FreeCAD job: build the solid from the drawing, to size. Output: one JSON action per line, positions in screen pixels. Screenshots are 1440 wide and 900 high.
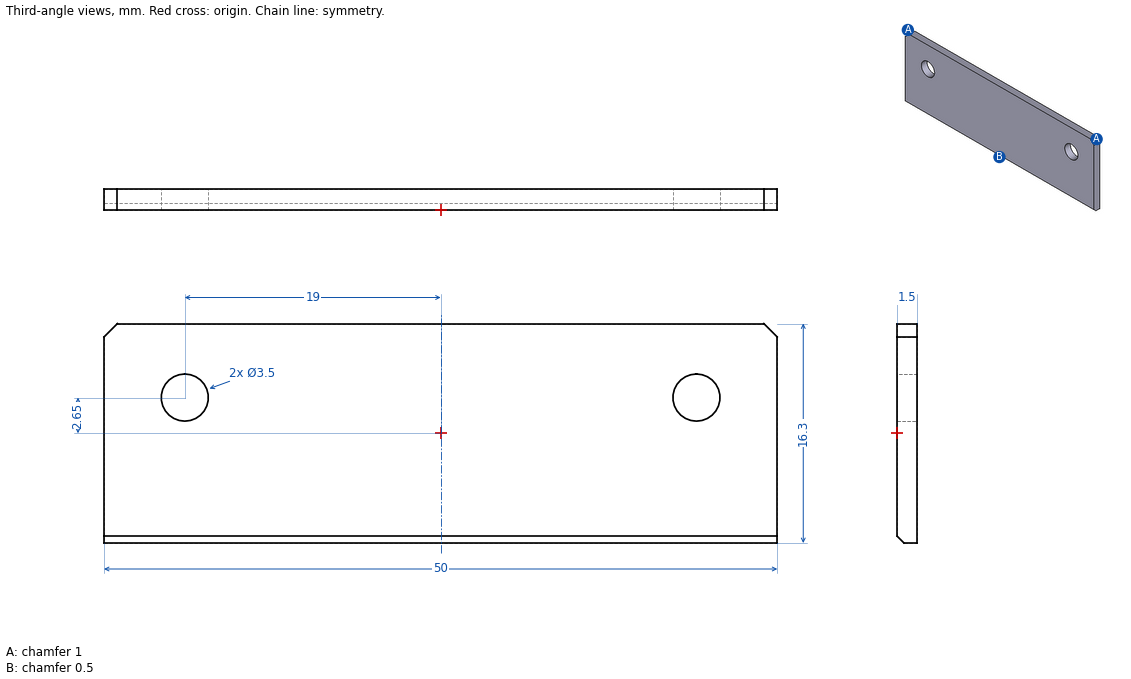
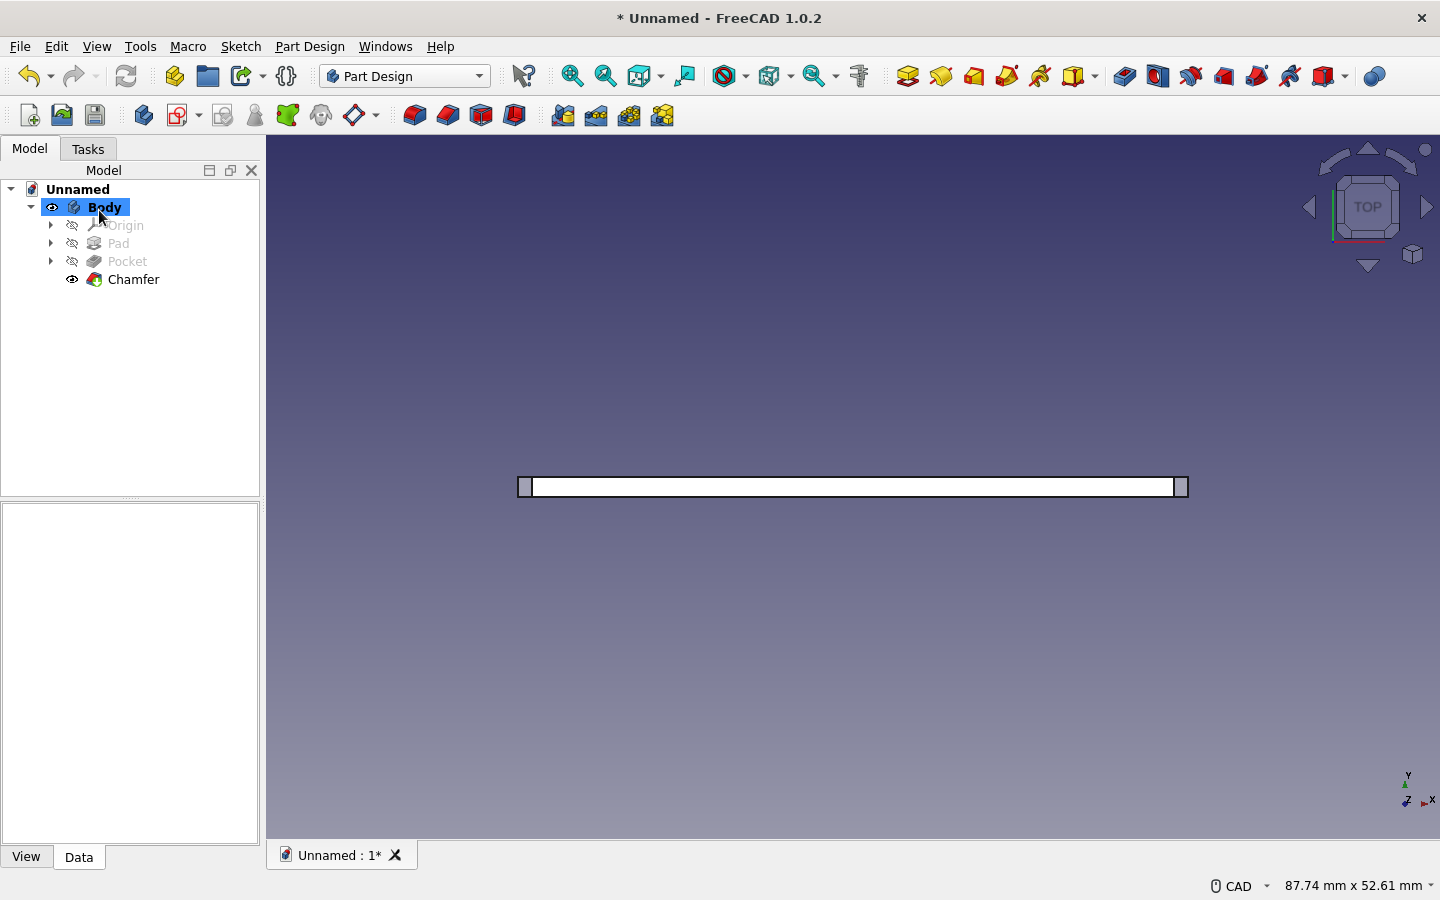
{"action": "key", "text": "1"}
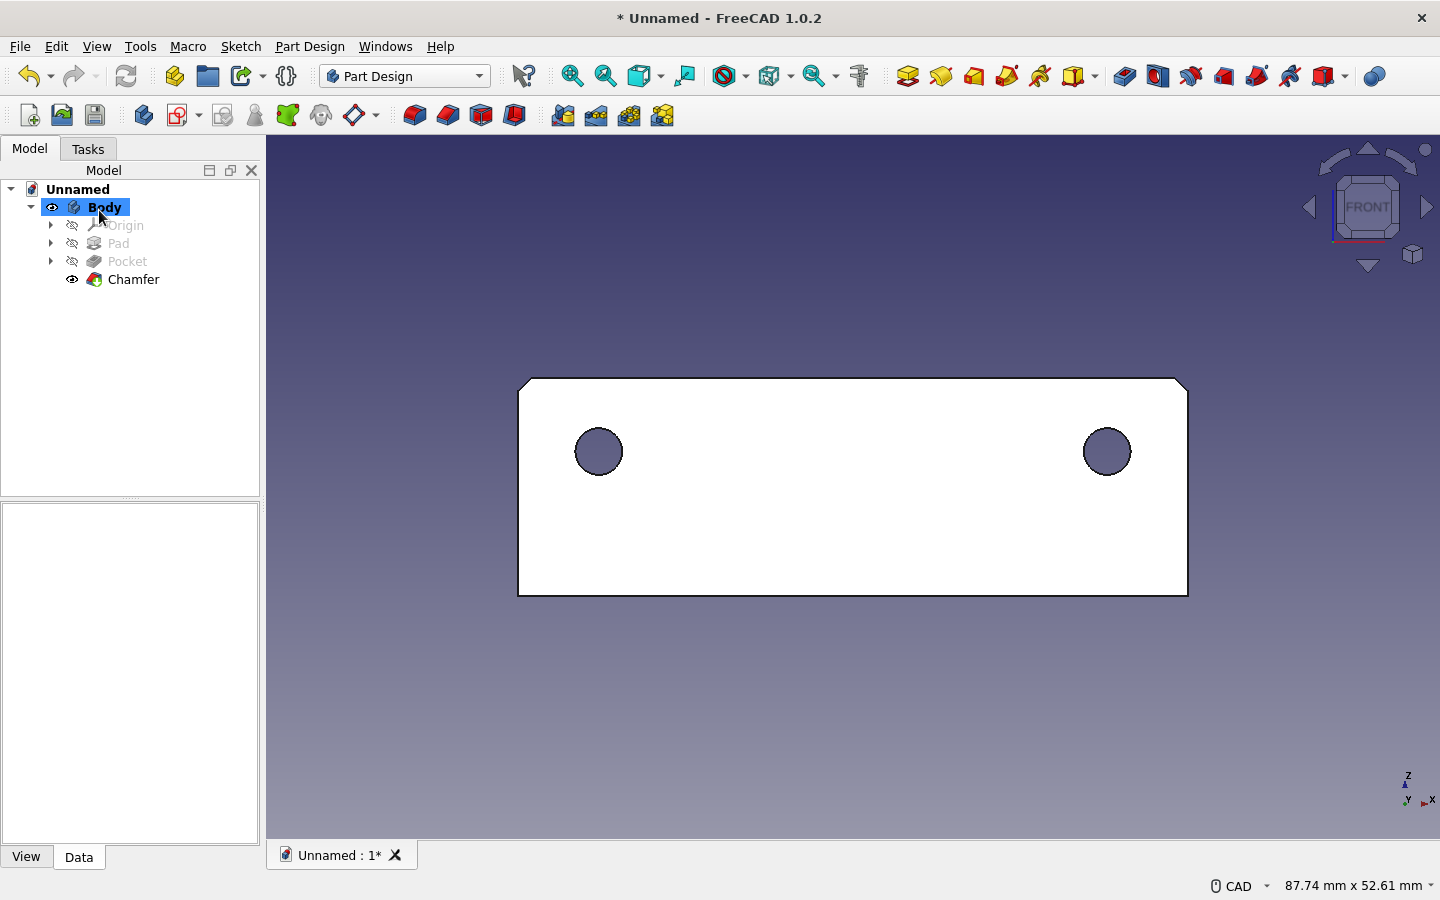
{"action": "key", "text": "3"}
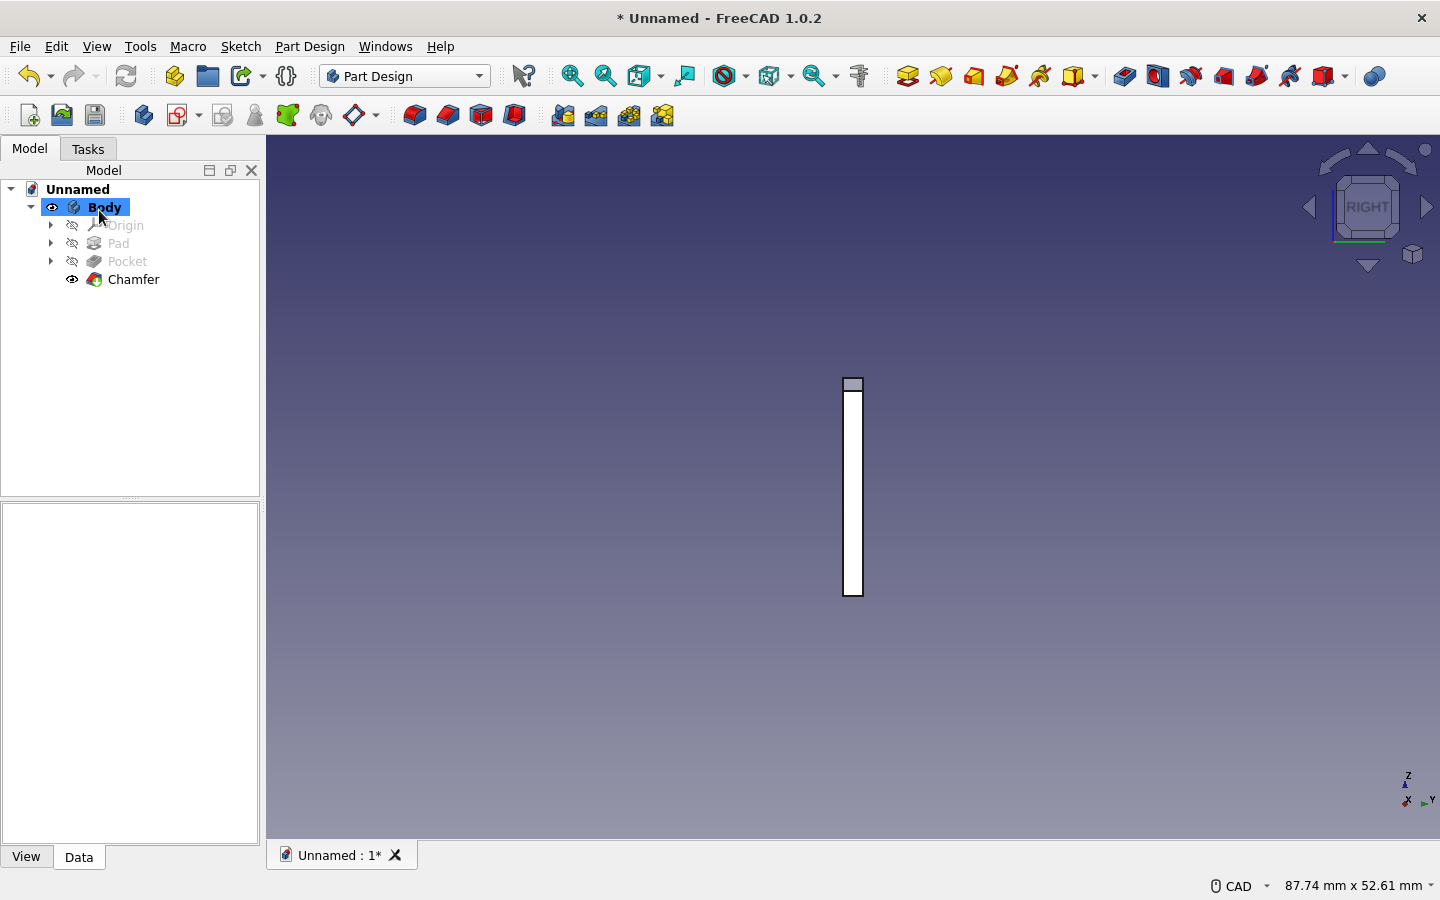
{"action": "key", "text": "v f"}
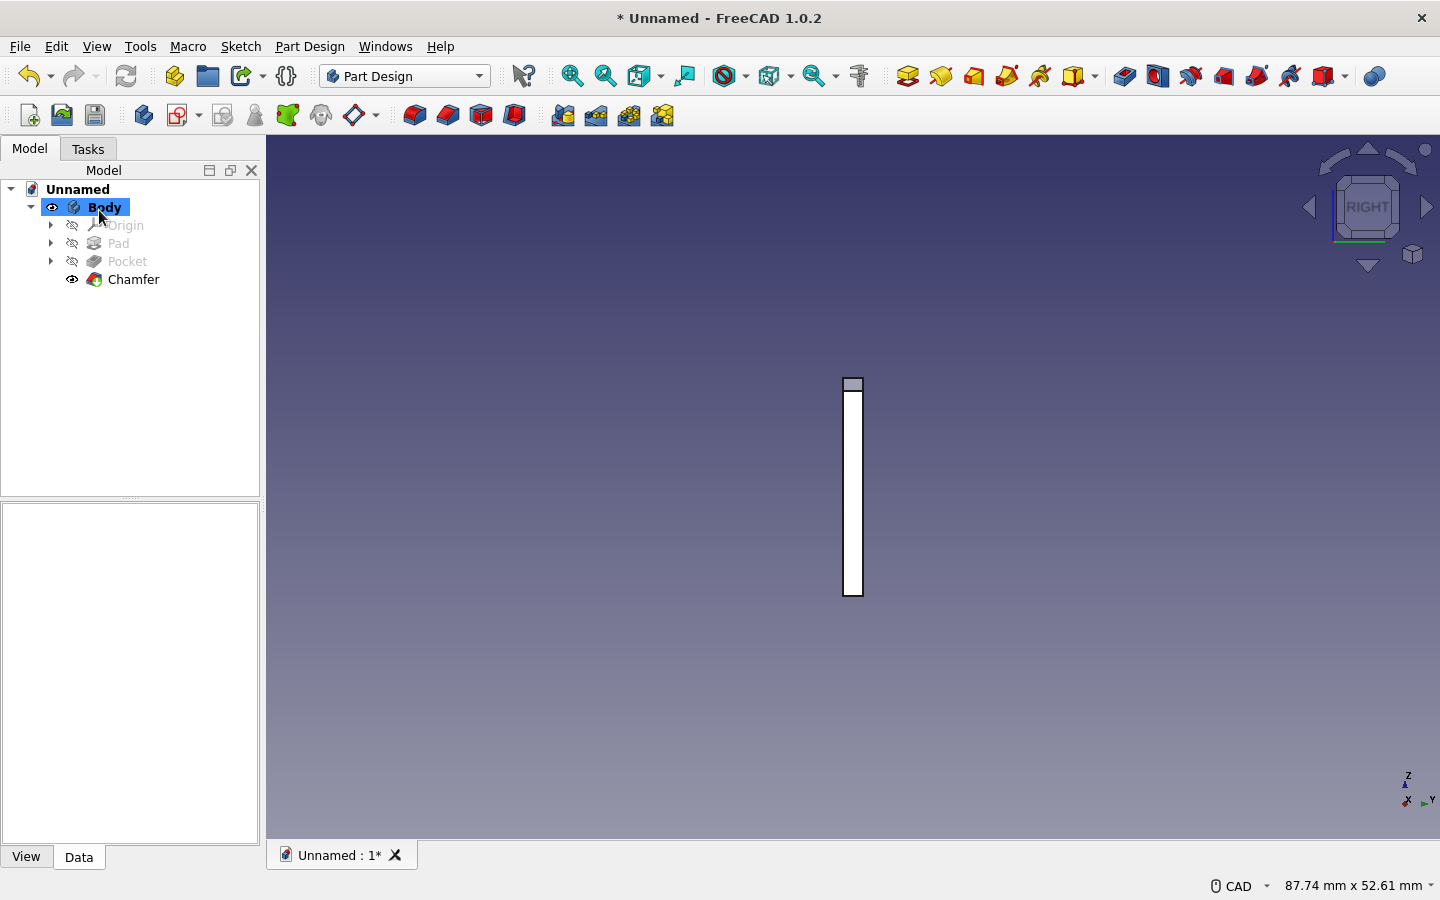
{"action": "key", "text": "5"}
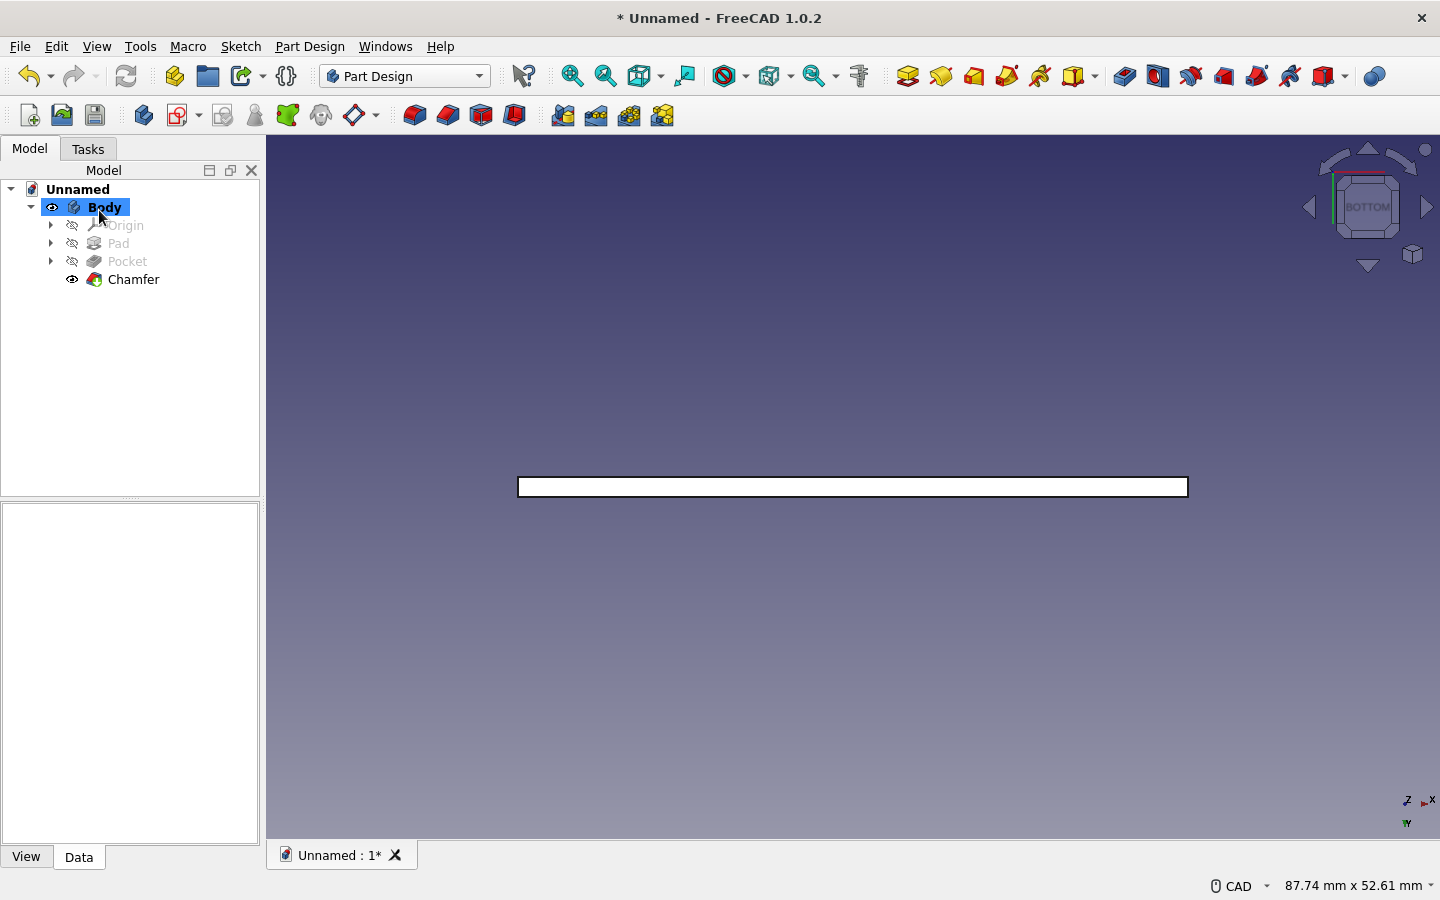
{"action": "left_click", "coordinate": [853, 476]}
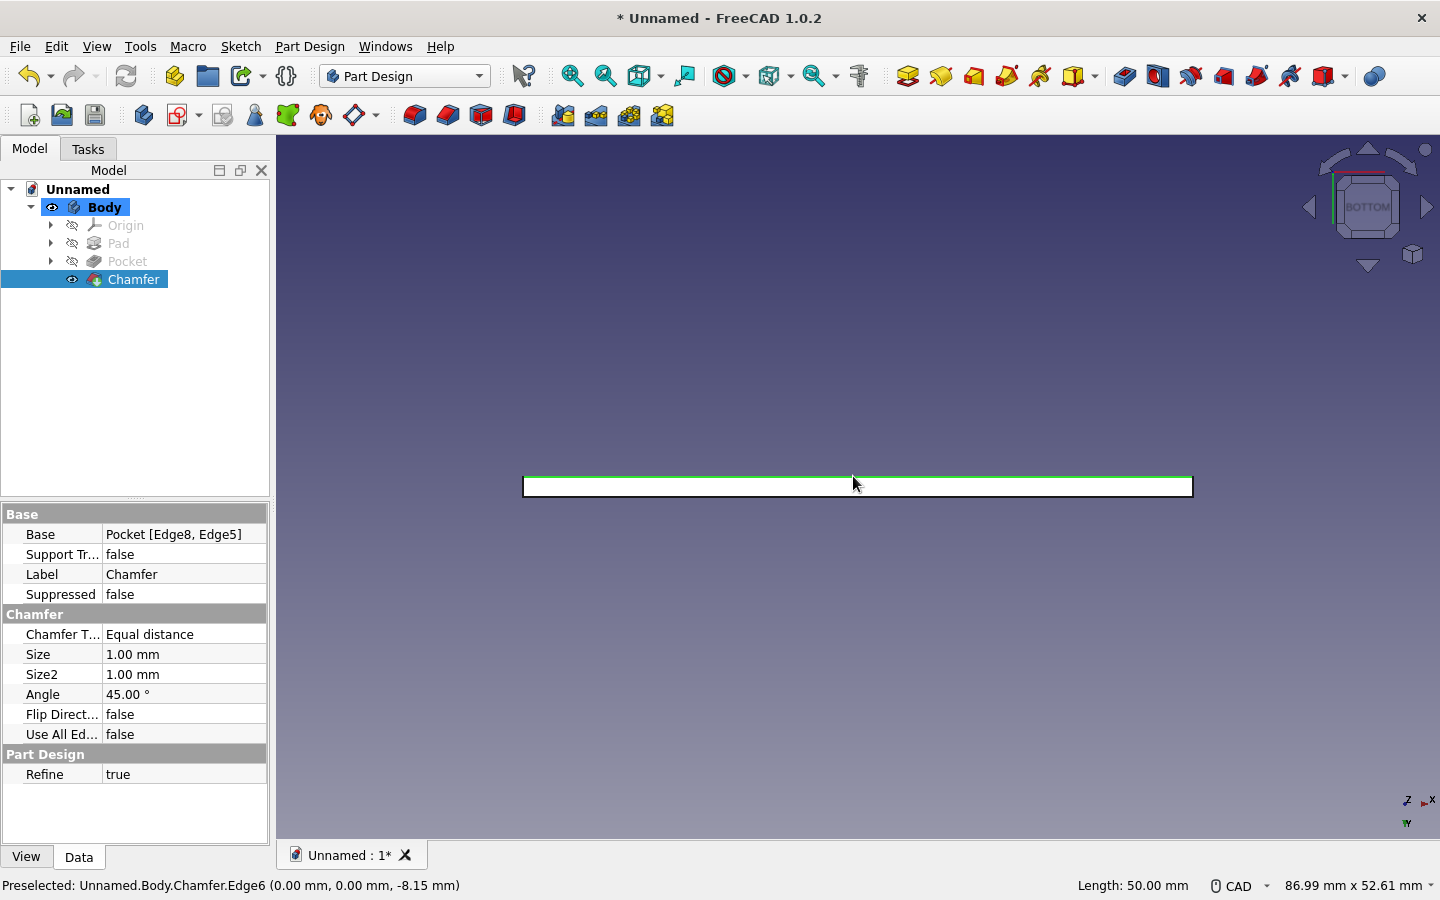
{"action": "left_click", "coordinate": [448, 116]}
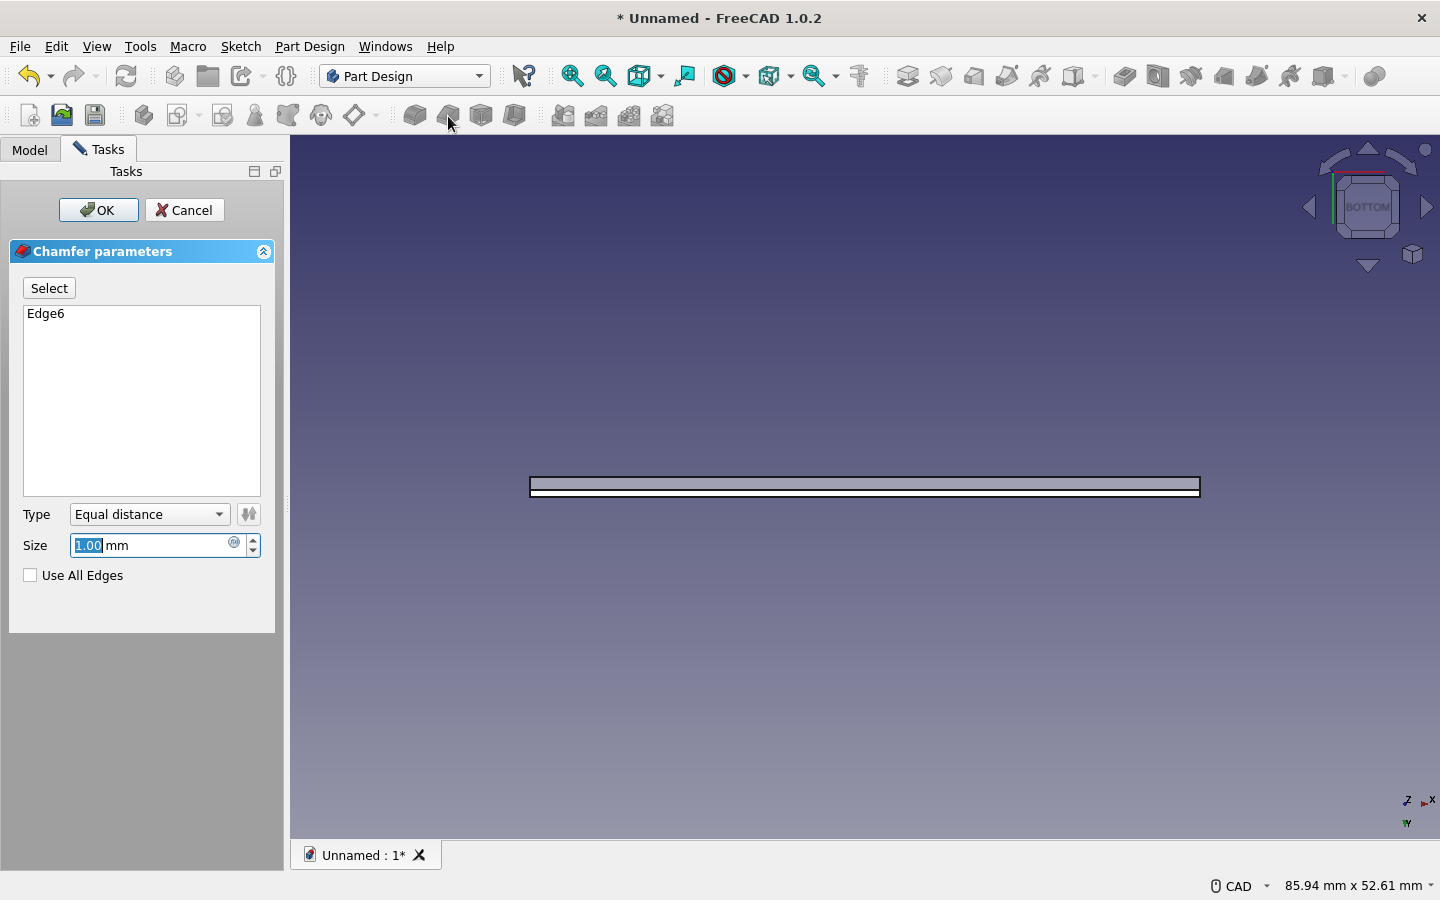
{"action": "type", "text": "0.5"}
{"action": "key", "text": "Tab"}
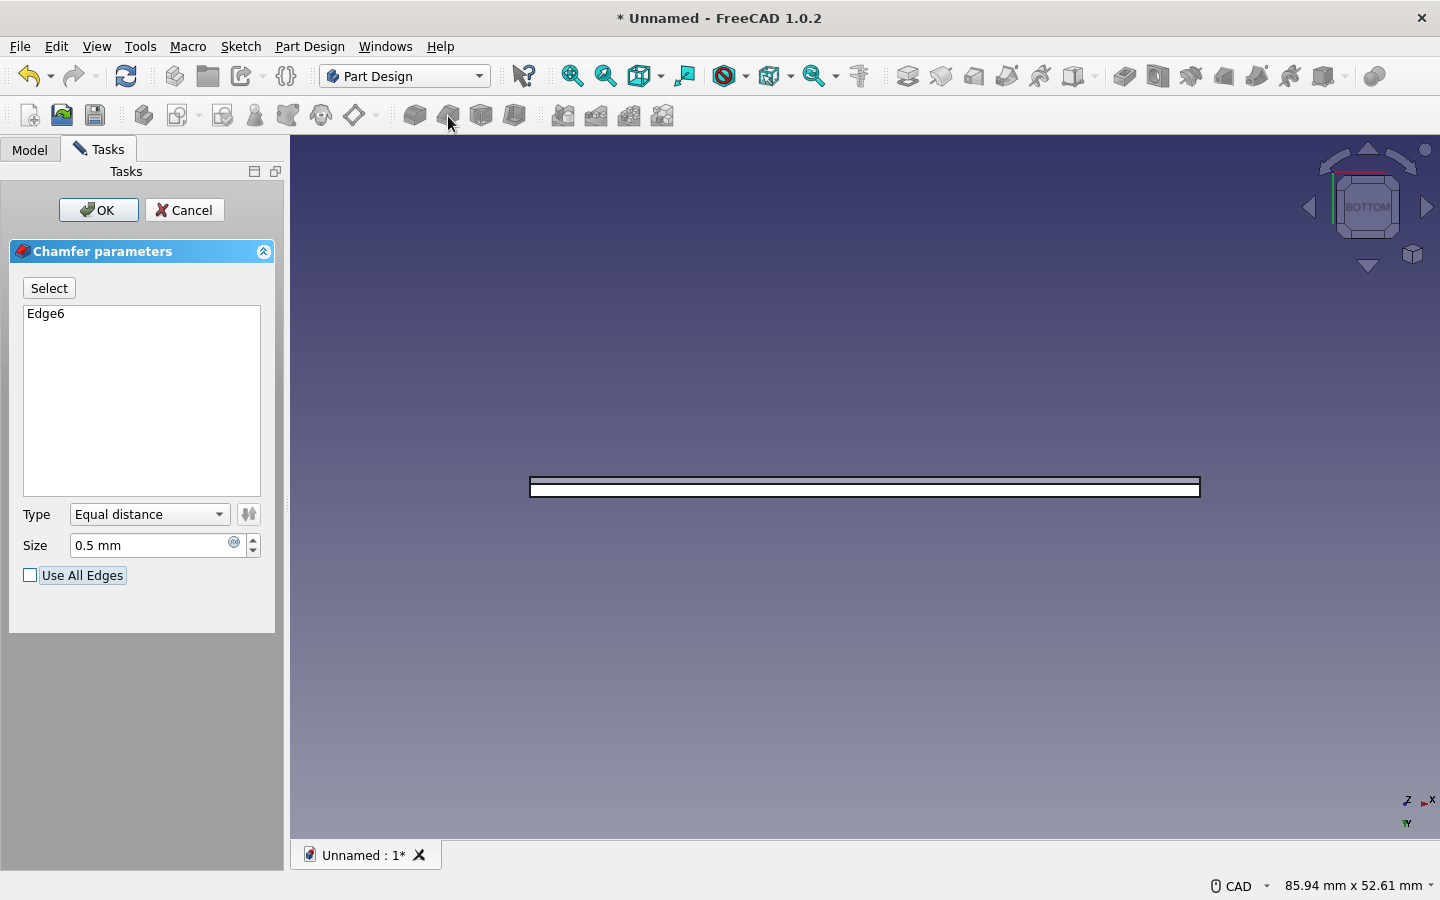
{"action": "left_click", "coordinate": [99, 210]}